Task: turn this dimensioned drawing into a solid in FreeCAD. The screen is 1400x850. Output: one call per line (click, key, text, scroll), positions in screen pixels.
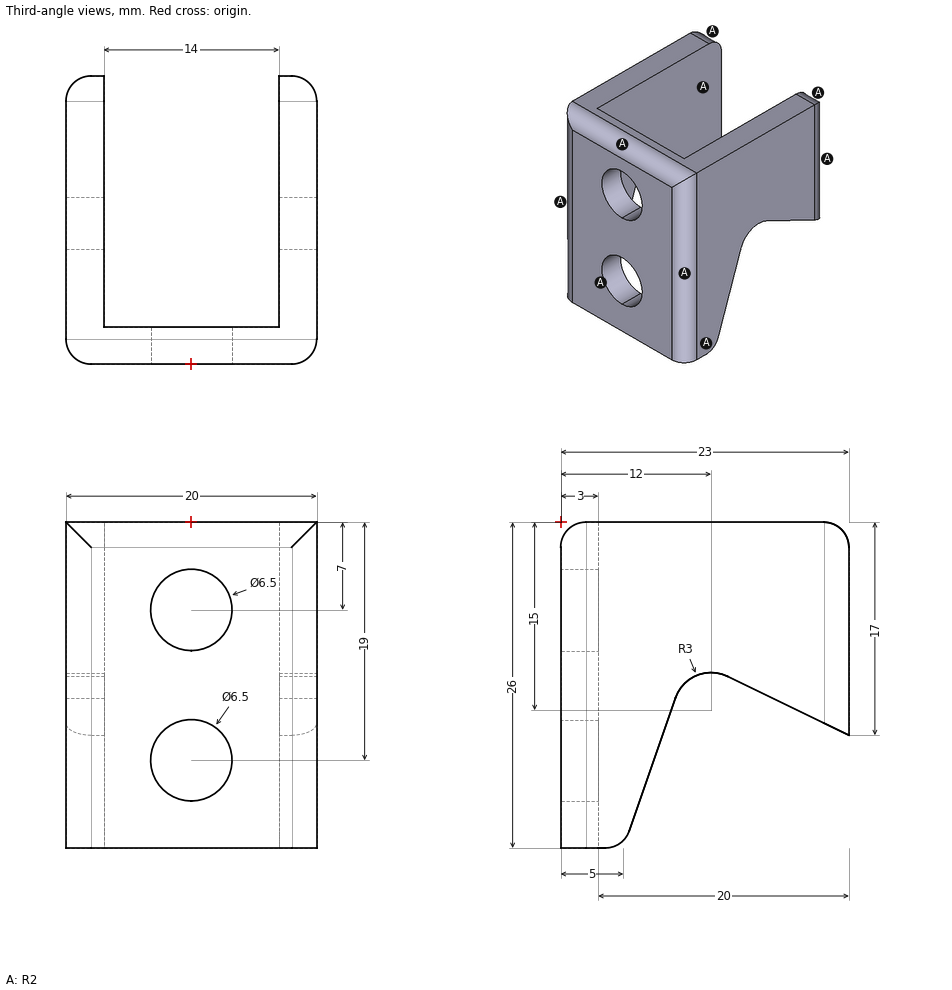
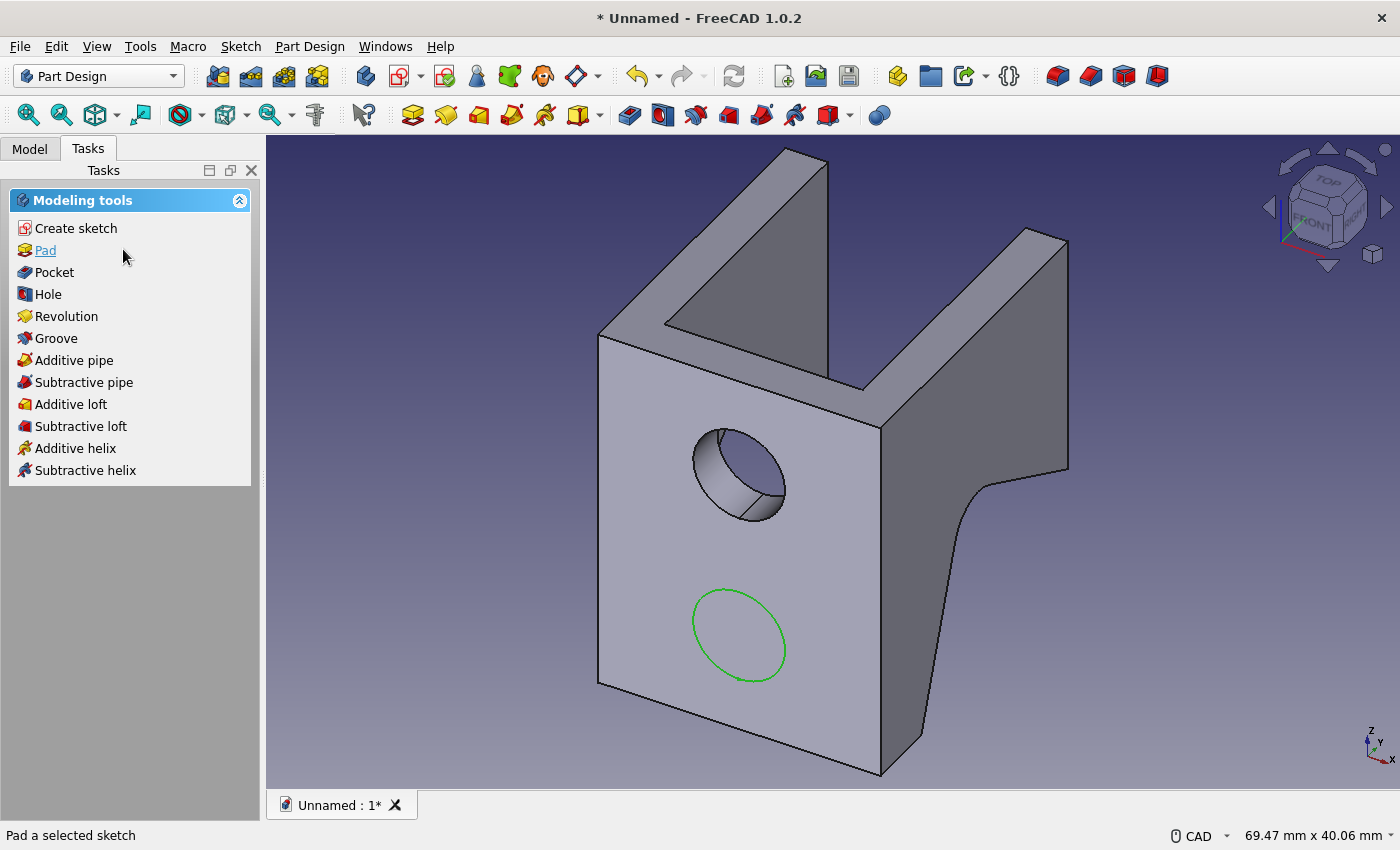
click(630, 116)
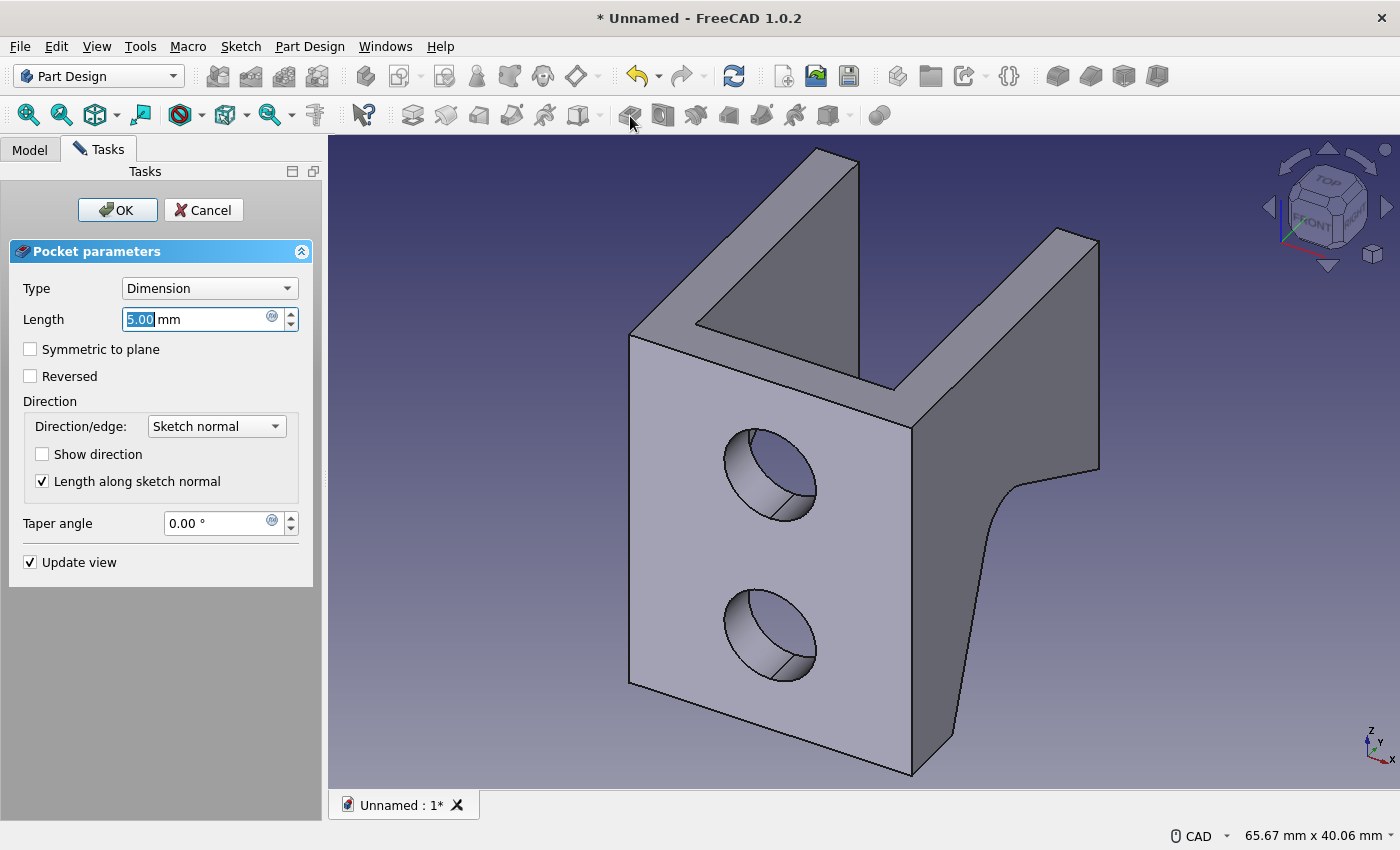
click(210, 288)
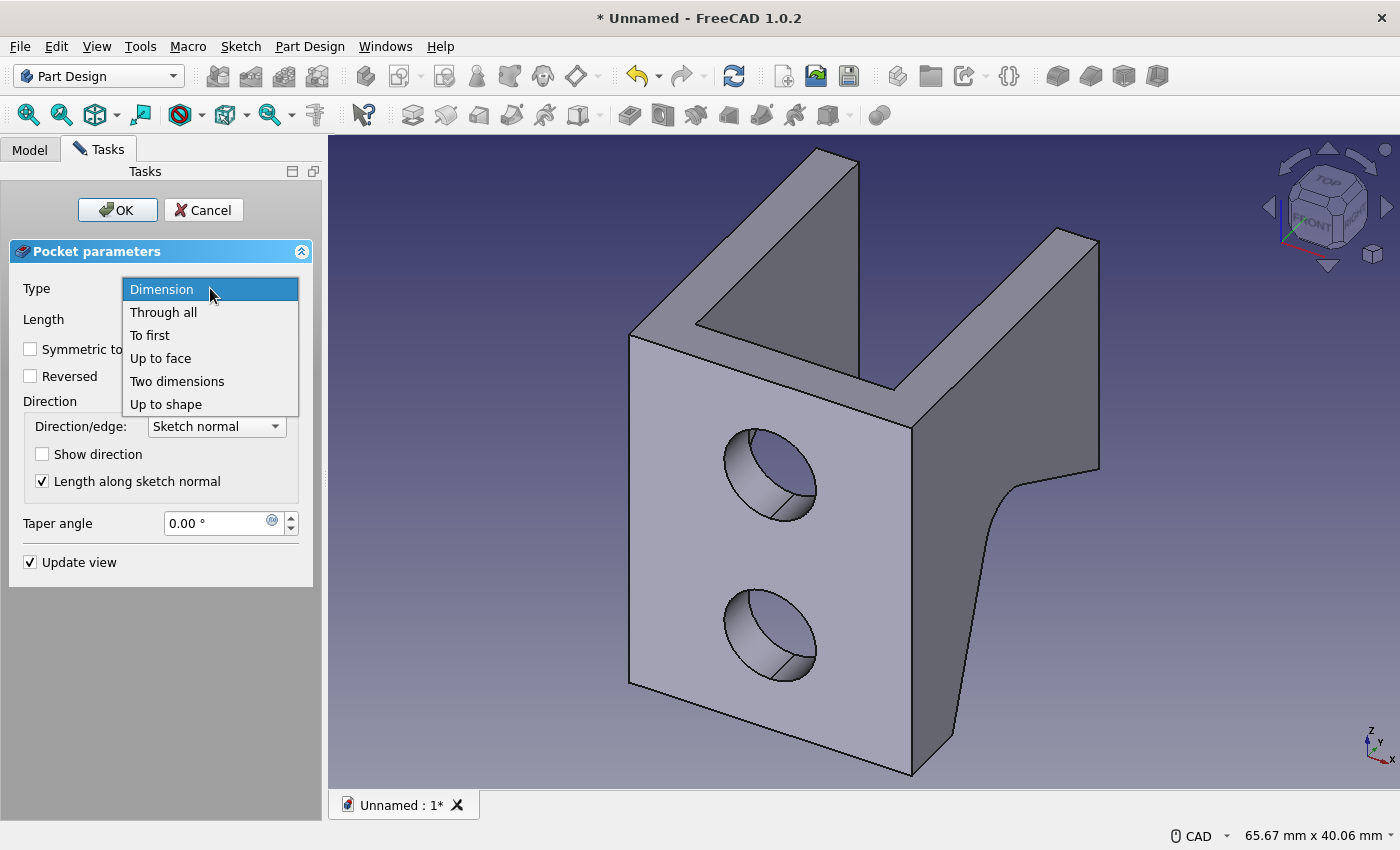
click(208, 336)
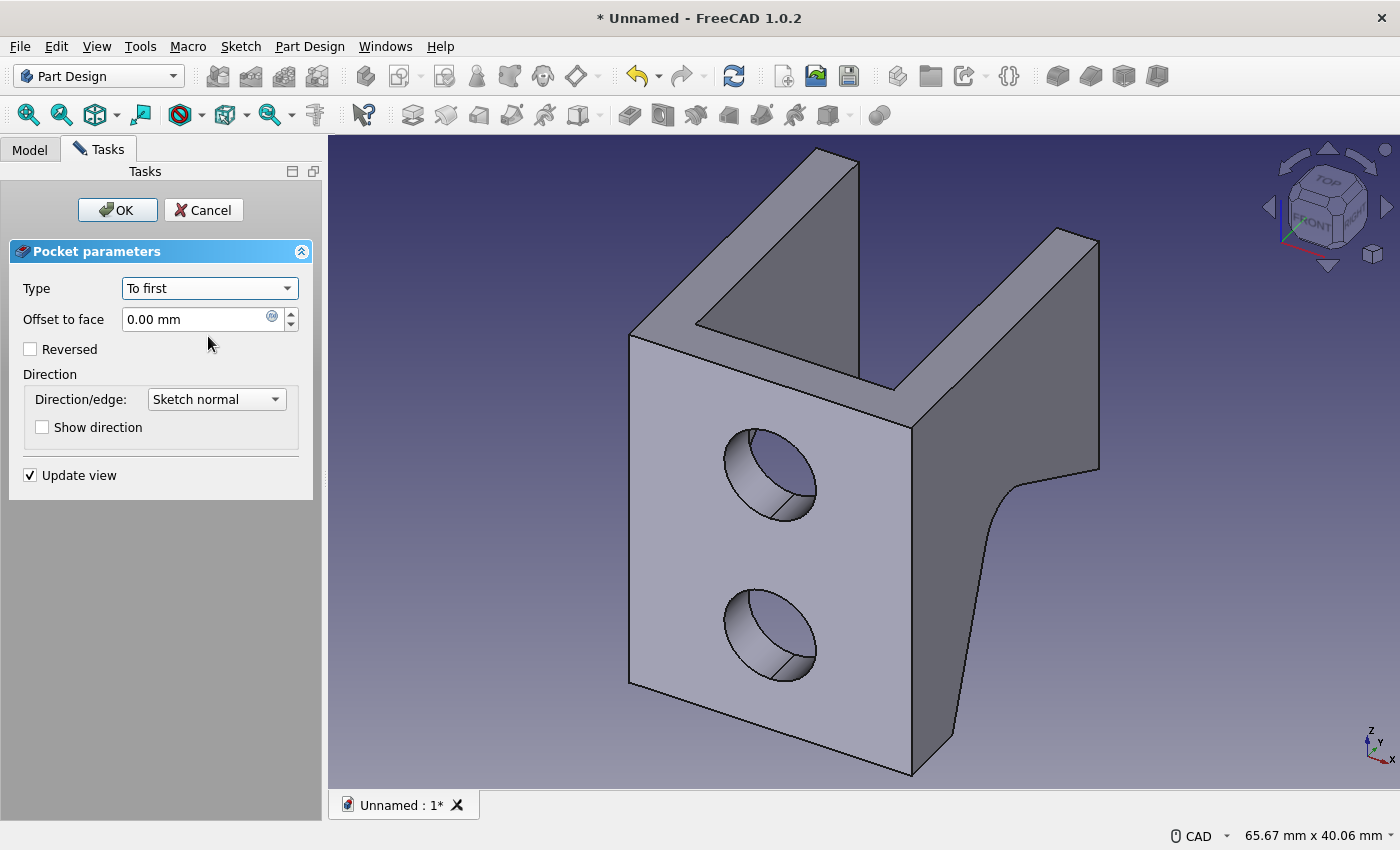
click(118, 210)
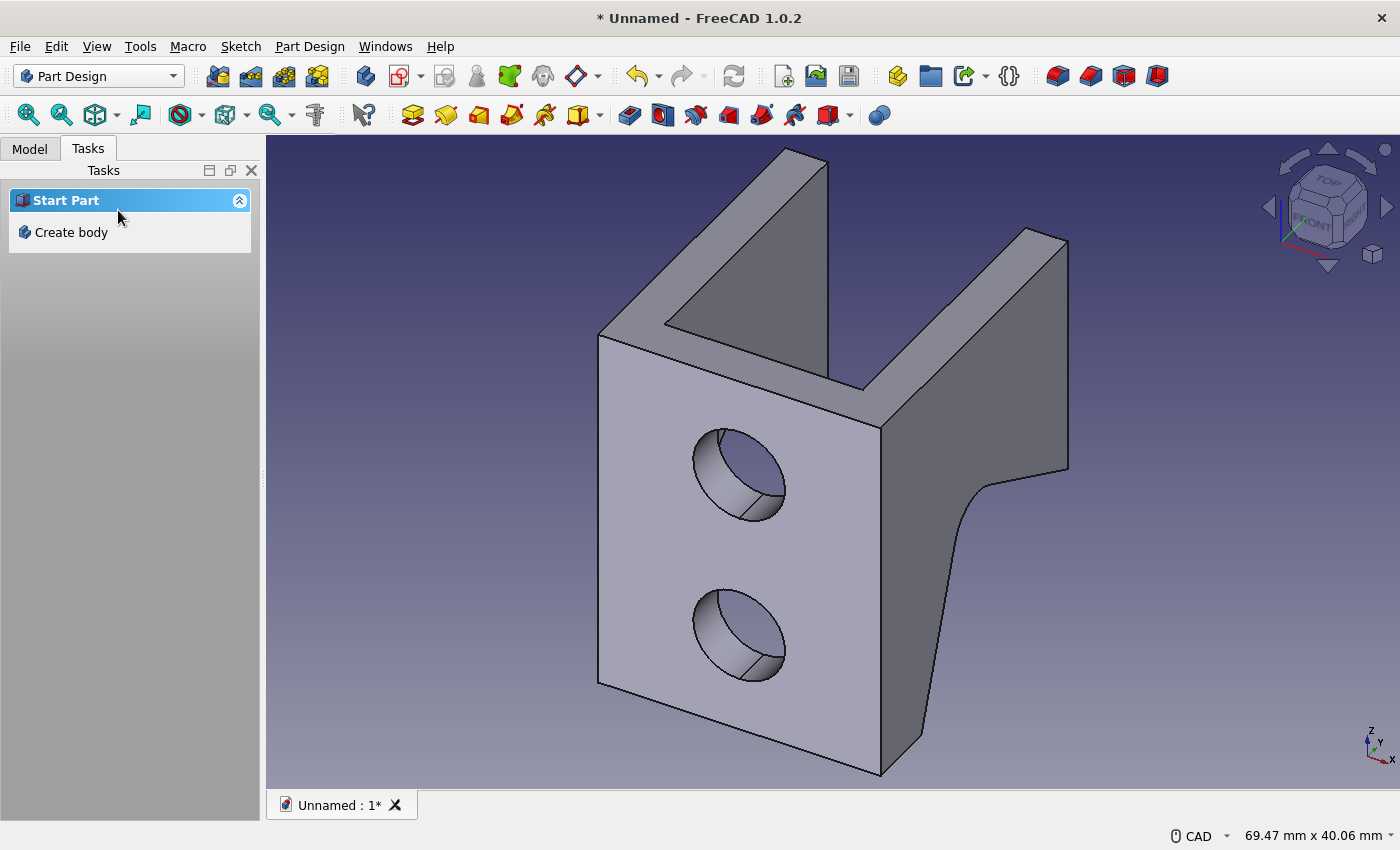
click(739, 380)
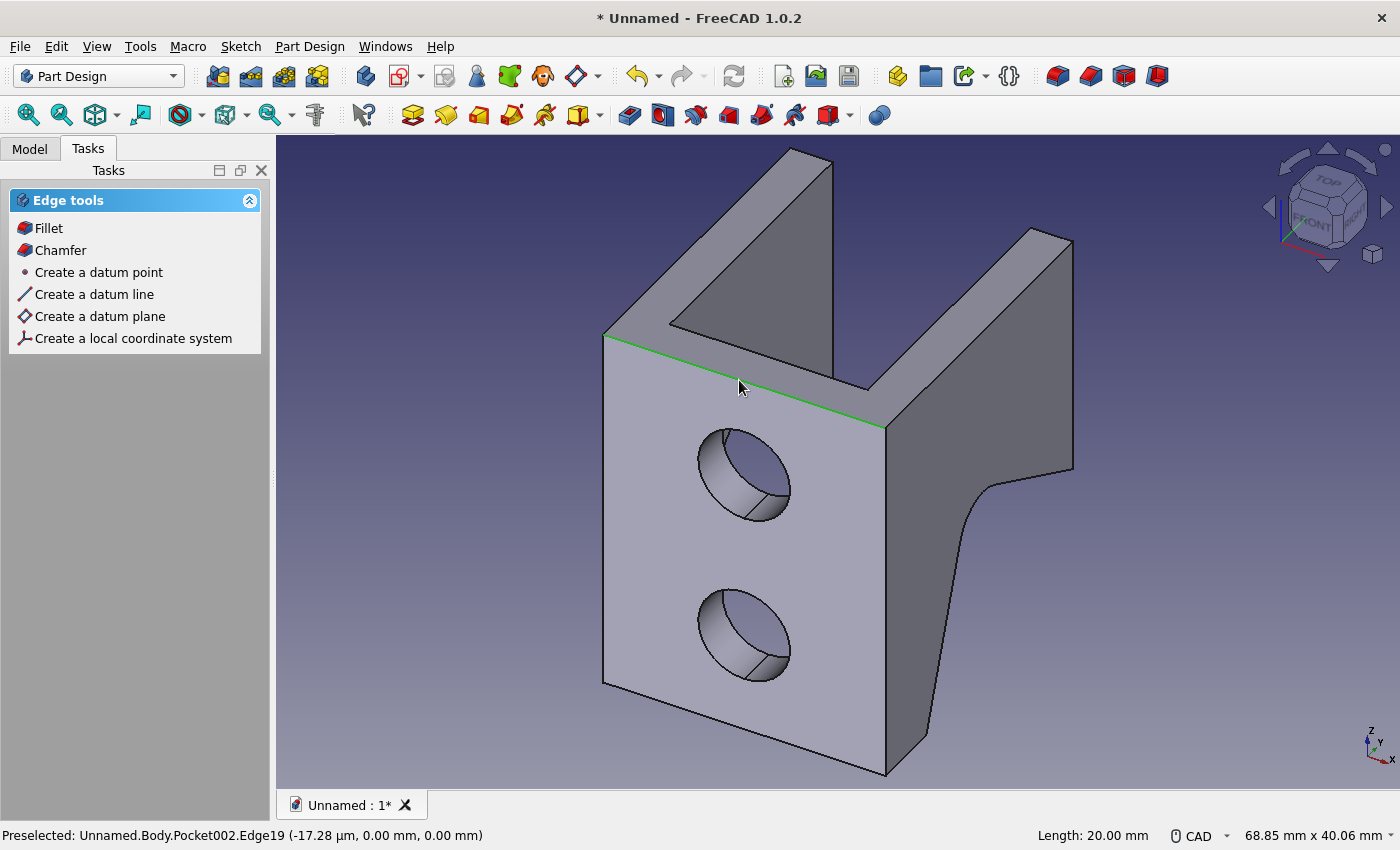
click(886, 601, ctrl)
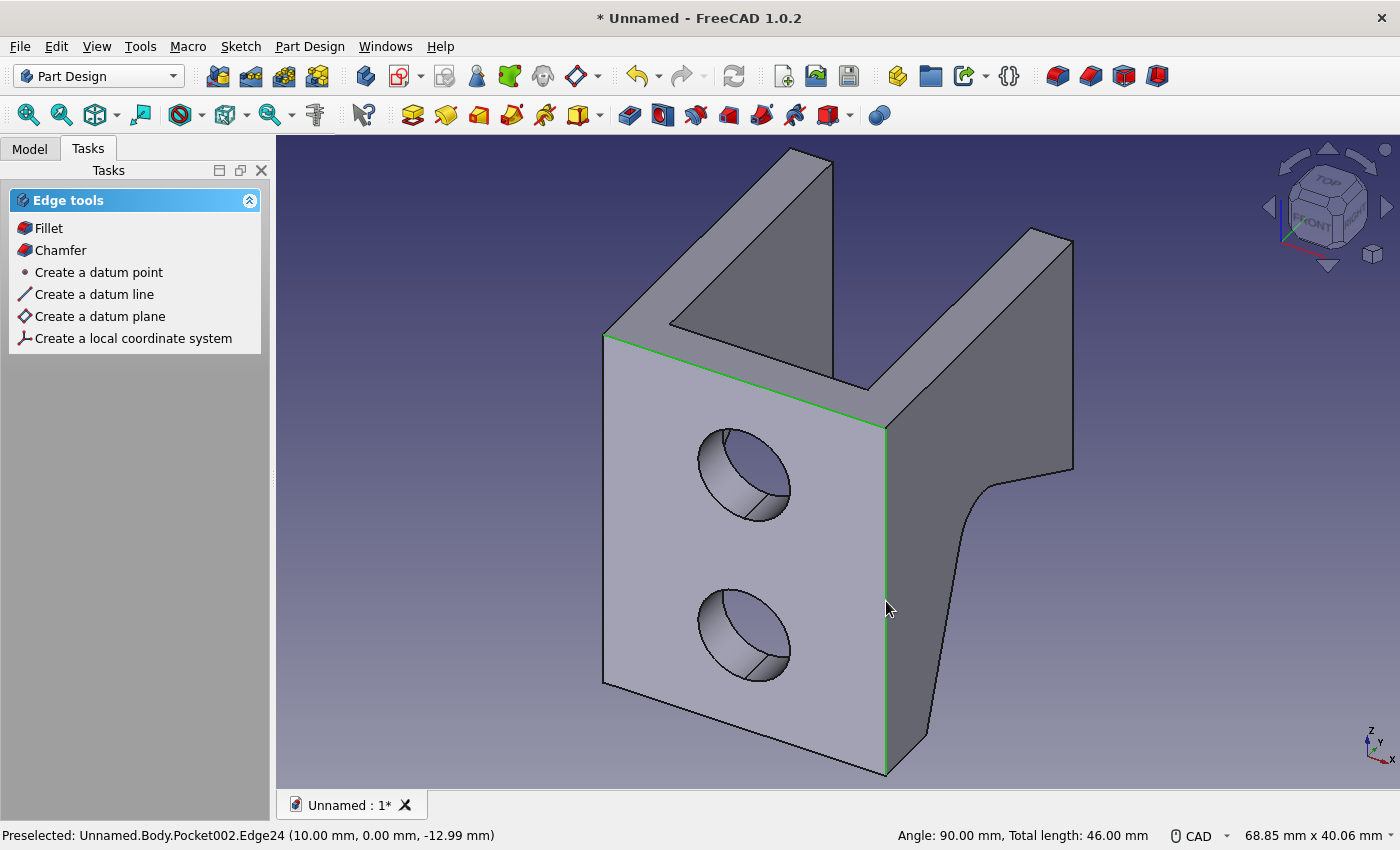
key(0)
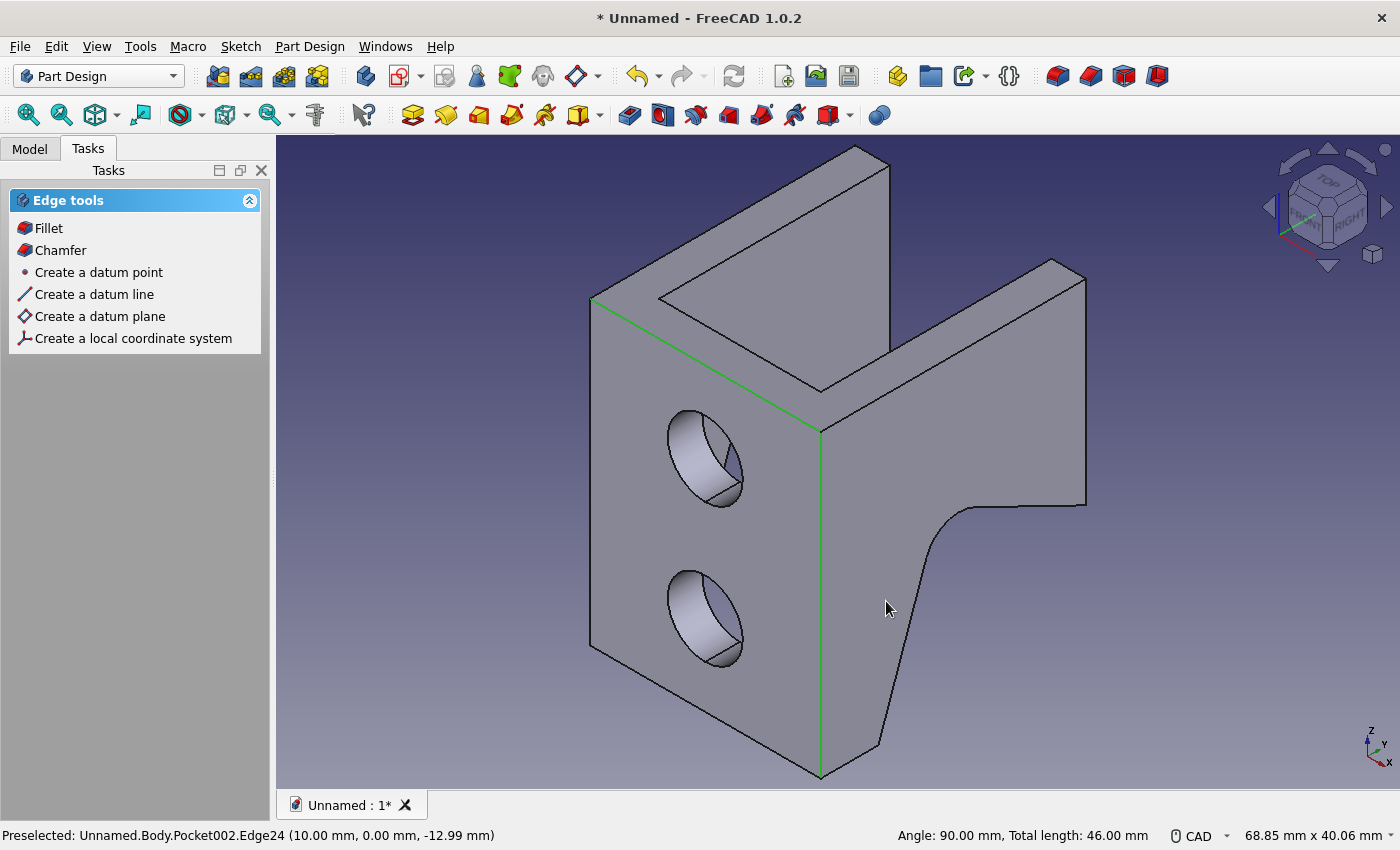
key(2)